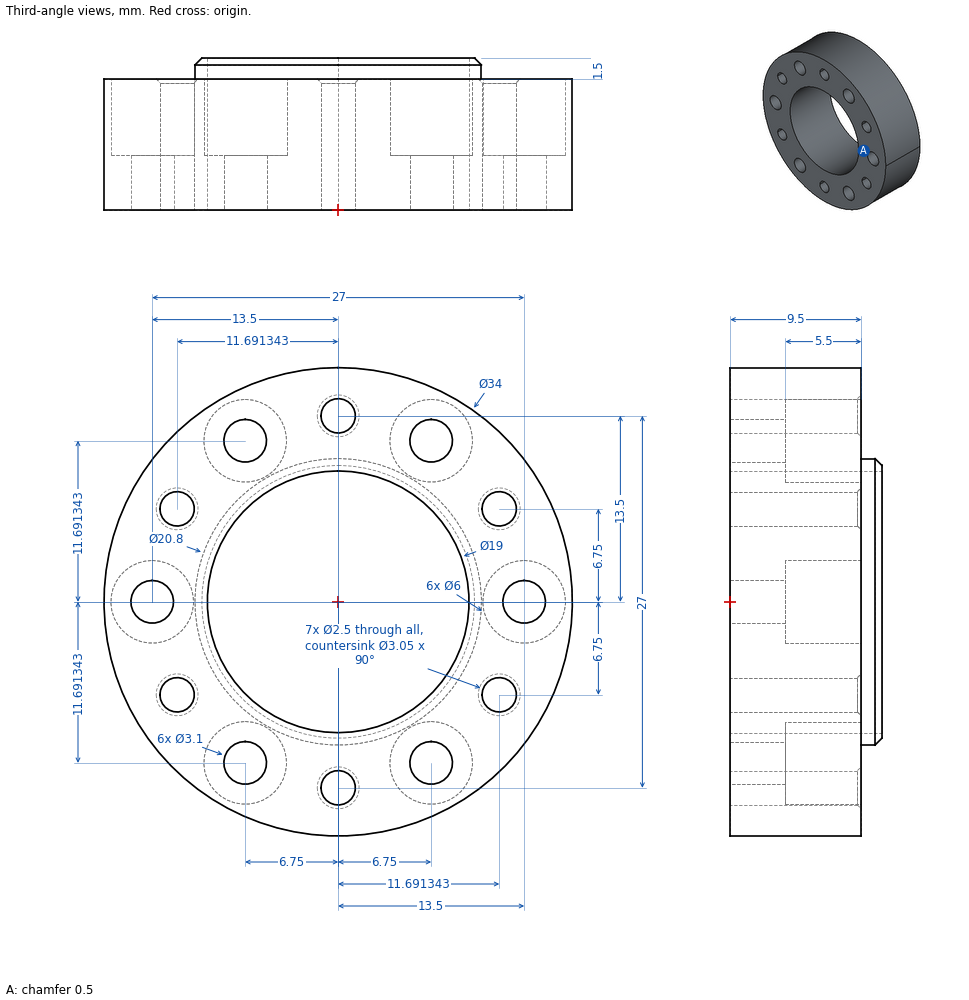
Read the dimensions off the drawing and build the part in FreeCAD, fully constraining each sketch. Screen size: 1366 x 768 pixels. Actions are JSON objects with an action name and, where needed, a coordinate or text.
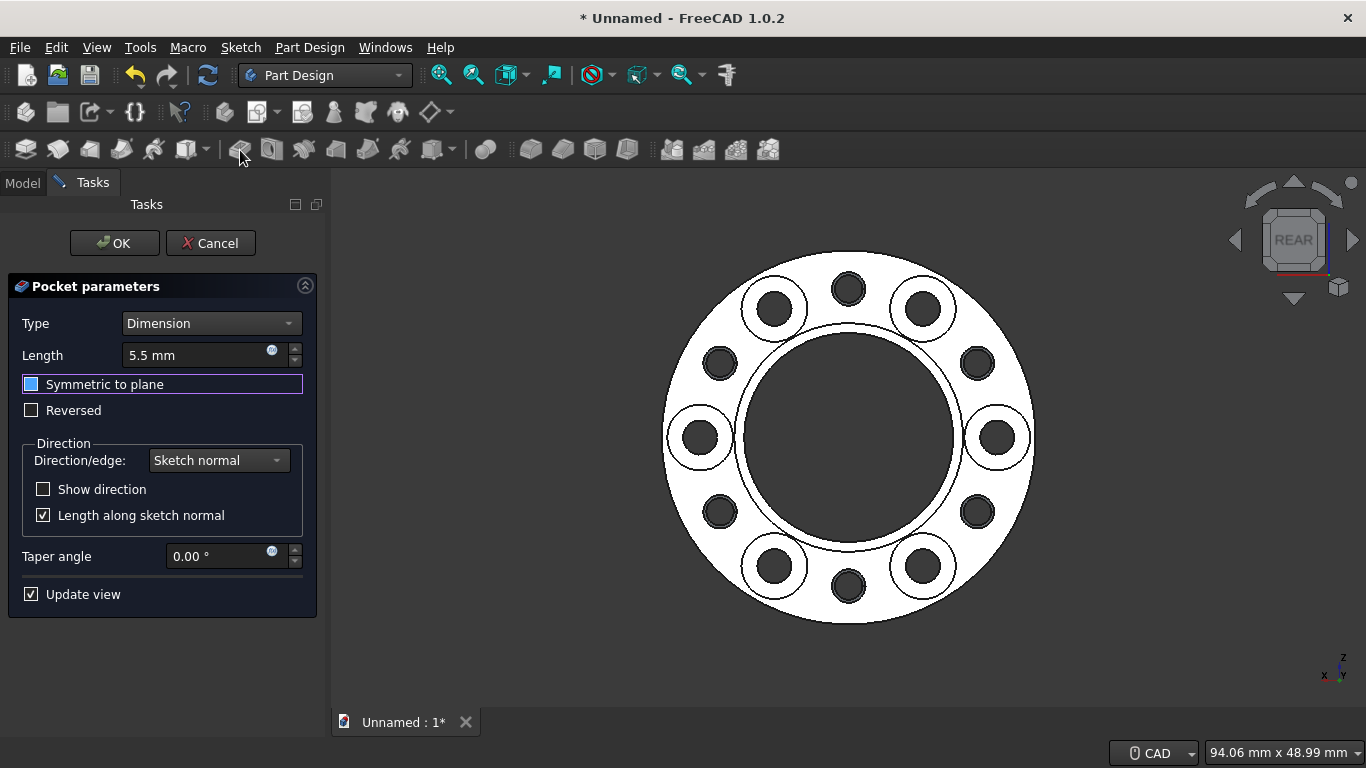
{"action": "left_click", "coordinate": [115, 243]}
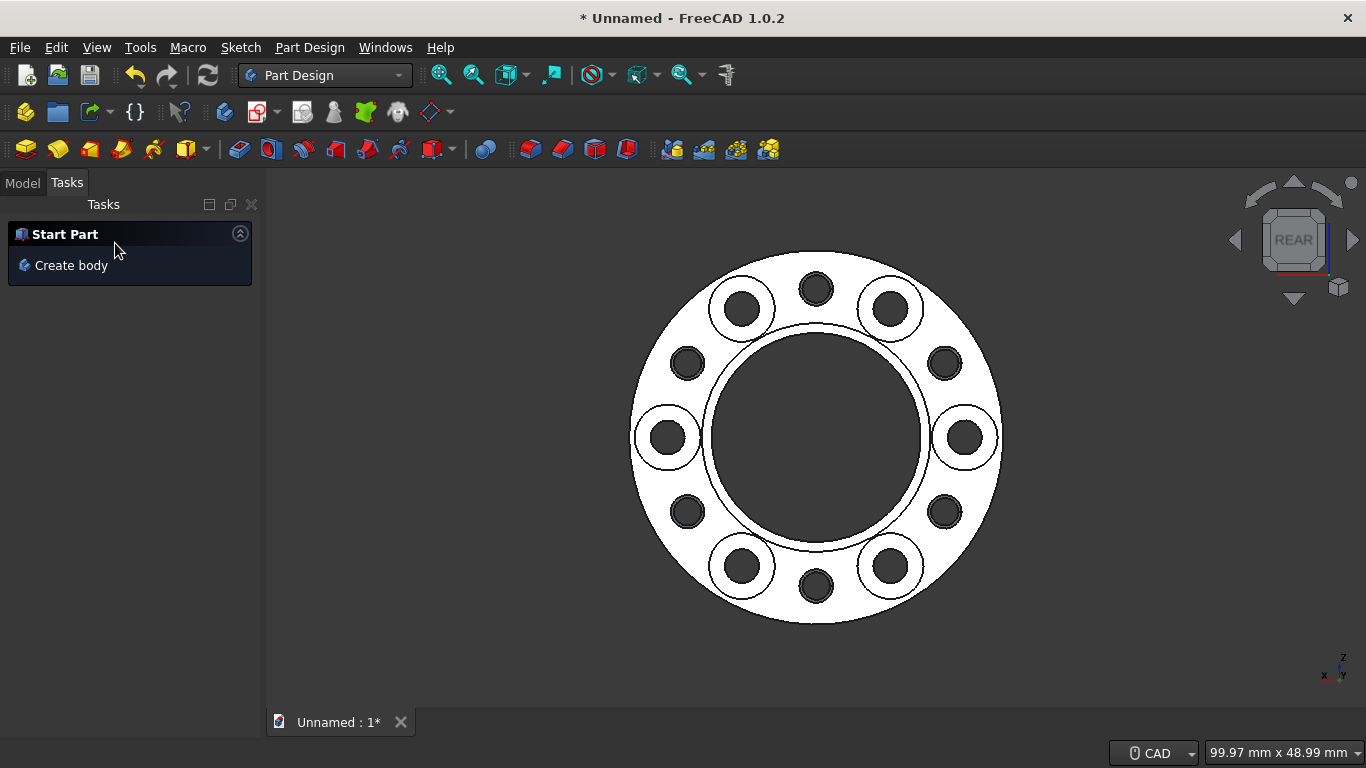
{"action": "left_click", "coordinate": [931, 437]}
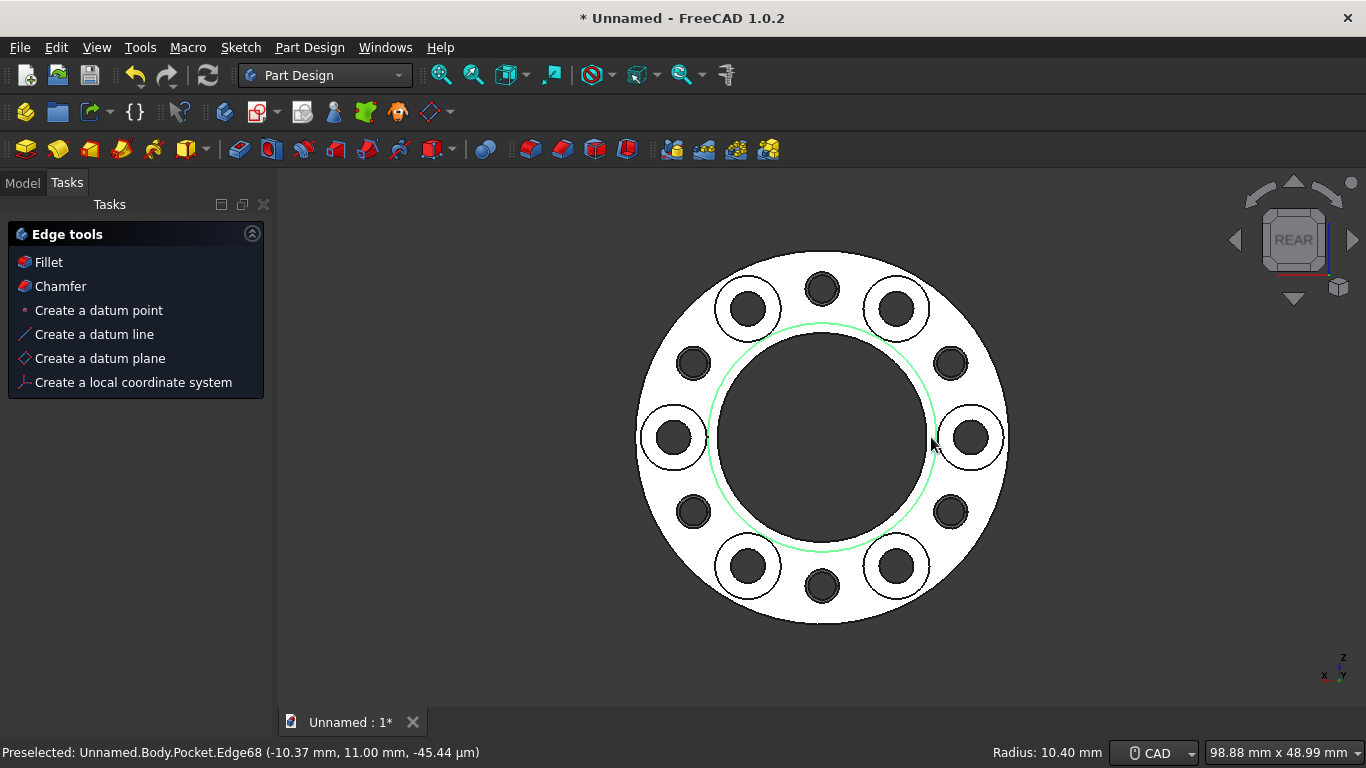
{"action": "left_click", "coordinate": [564, 150]}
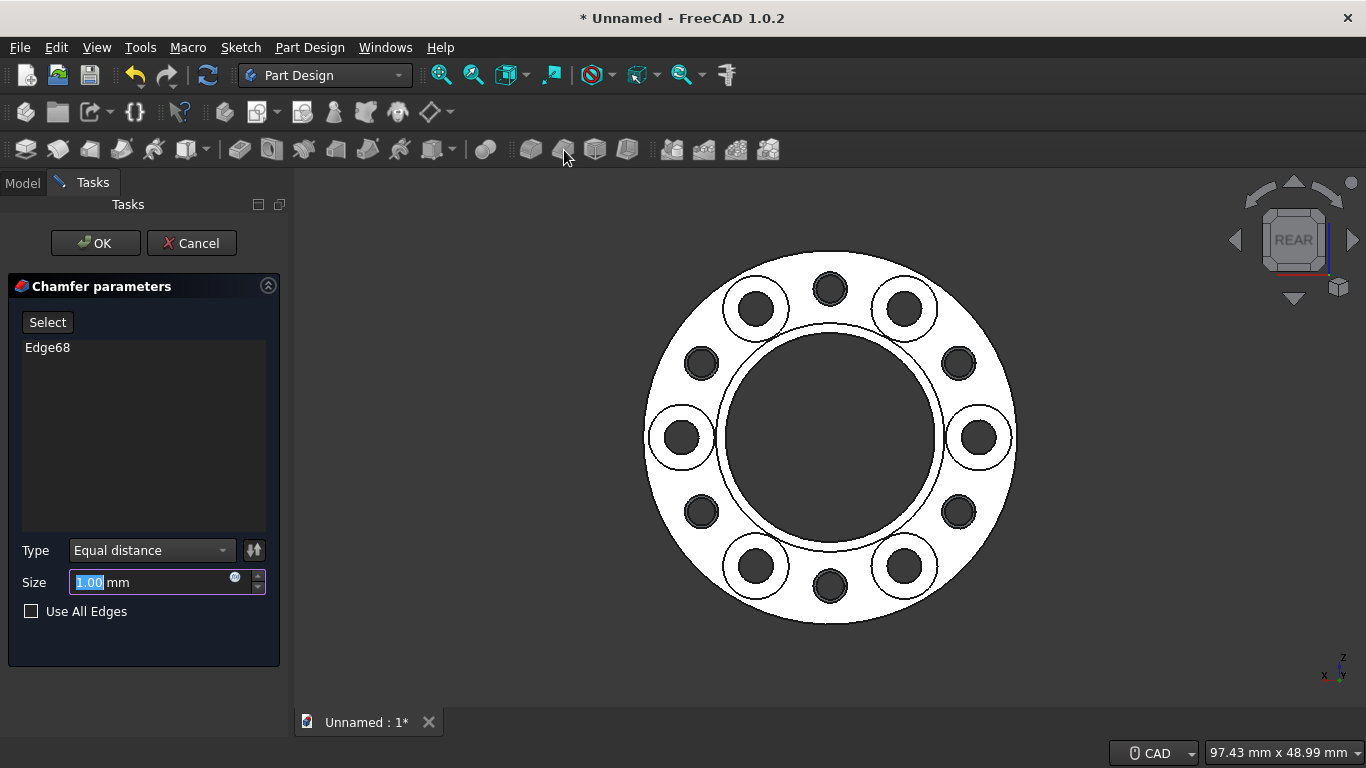
{"action": "type", "text": "0.5"}
{"action": "key", "text": "Tab"}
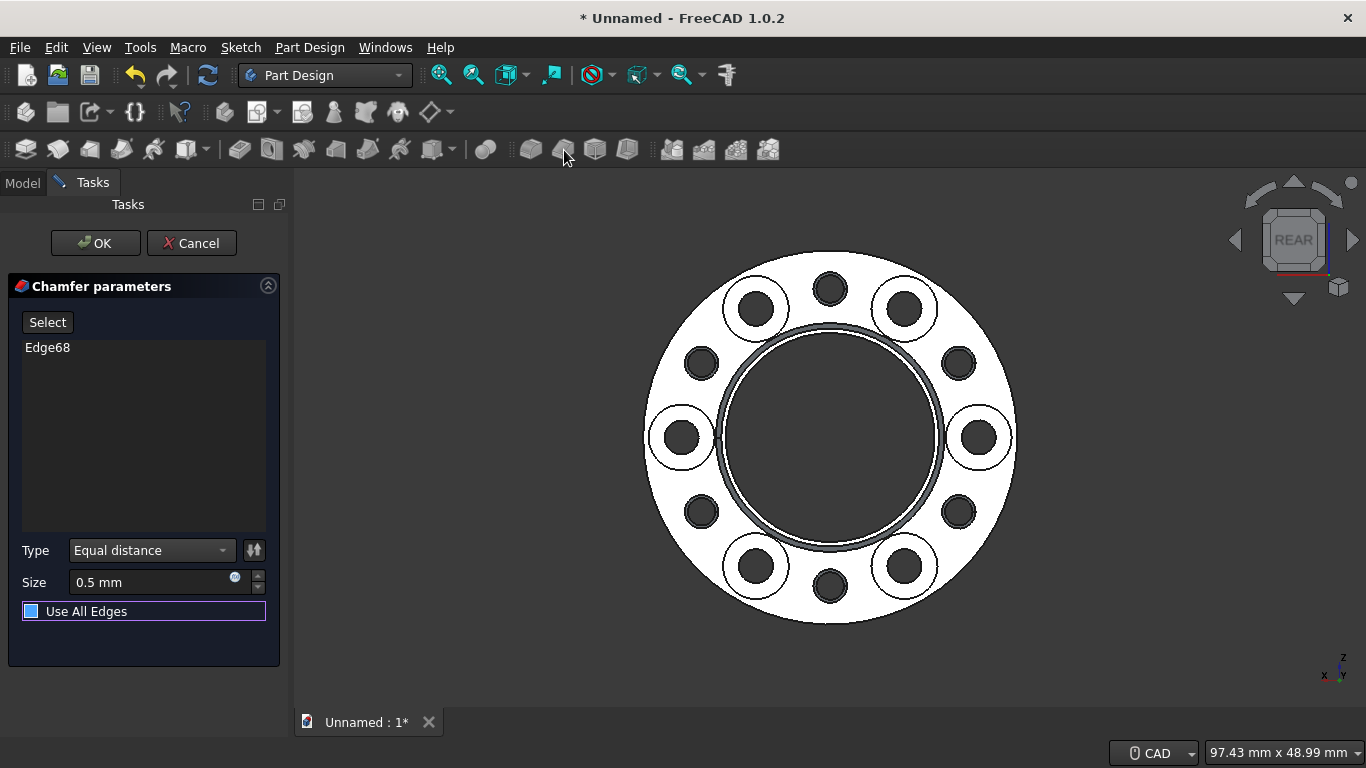
{"action": "left_click", "coordinate": [96, 243]}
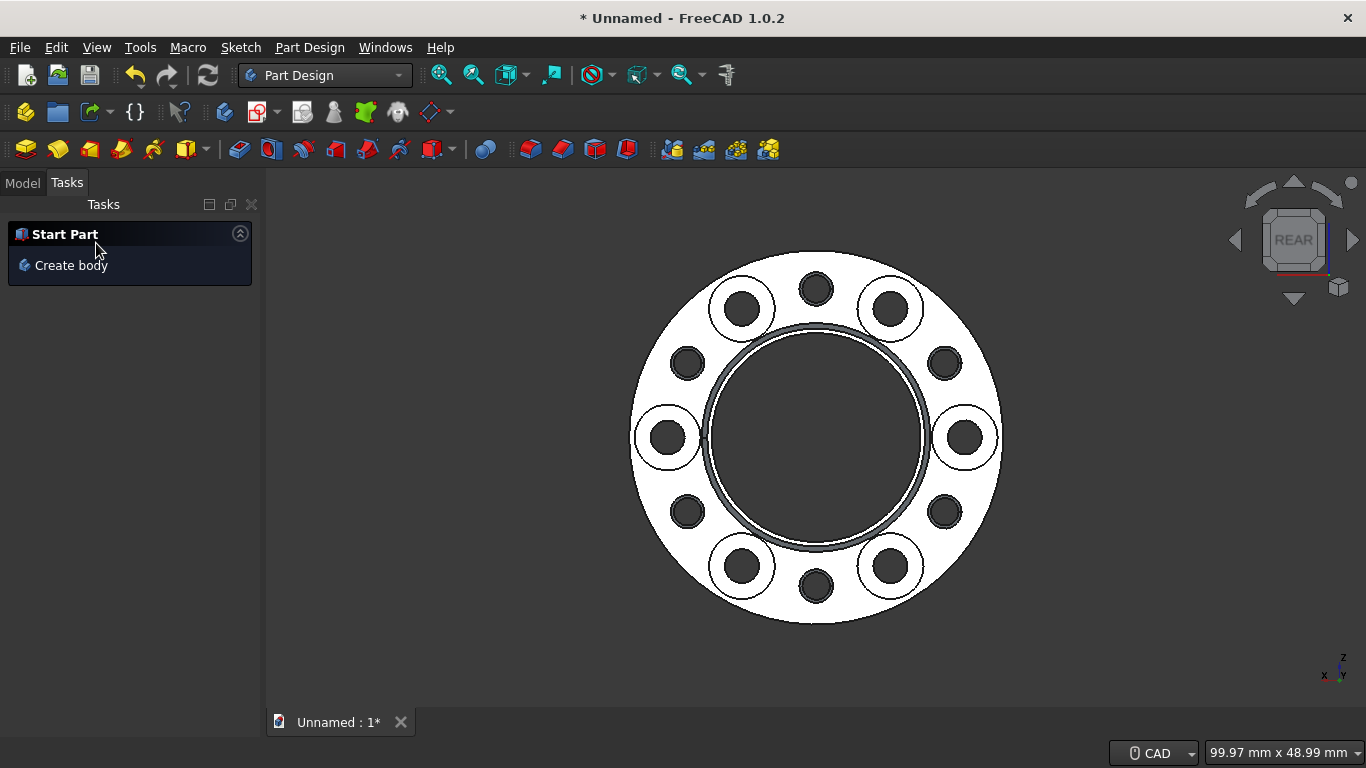
{"action": "key", "text": "0"}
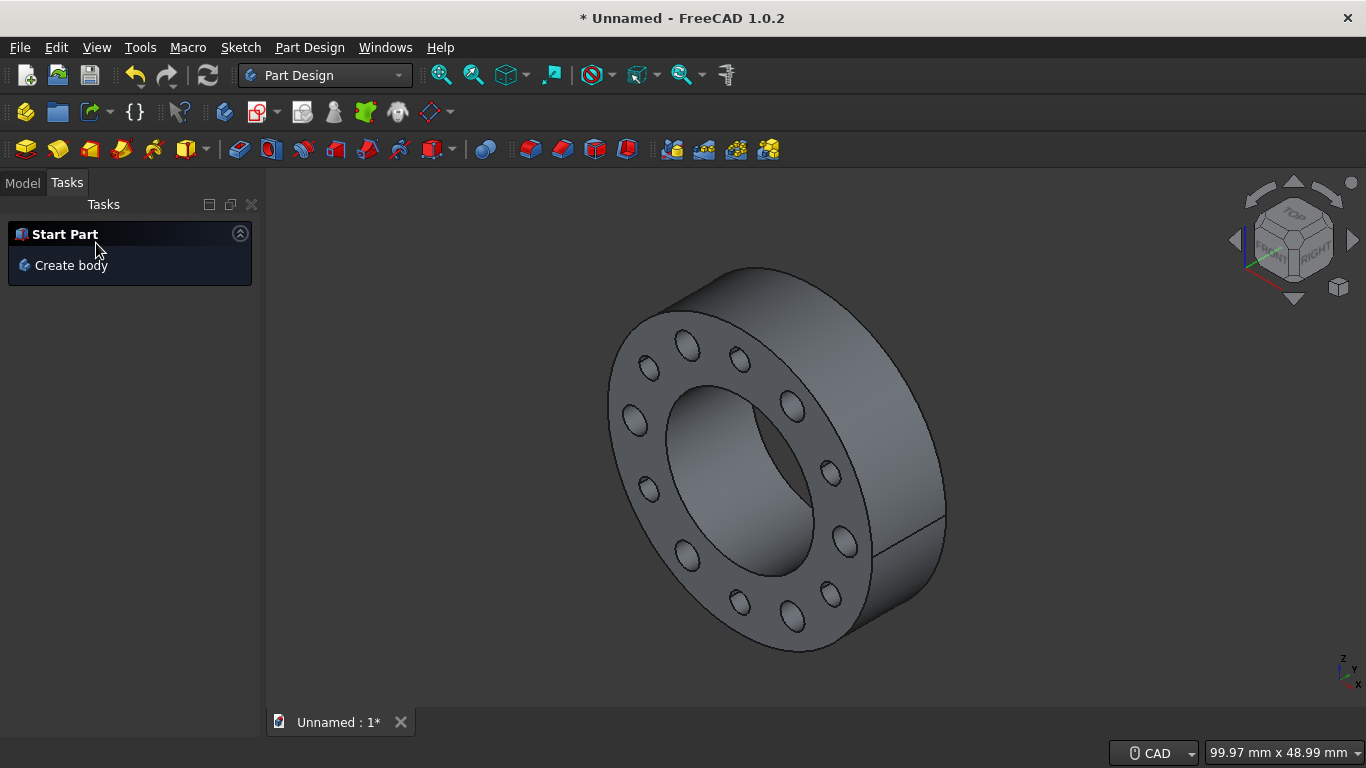
{"action": "left_click", "coordinate": [442, 76]}